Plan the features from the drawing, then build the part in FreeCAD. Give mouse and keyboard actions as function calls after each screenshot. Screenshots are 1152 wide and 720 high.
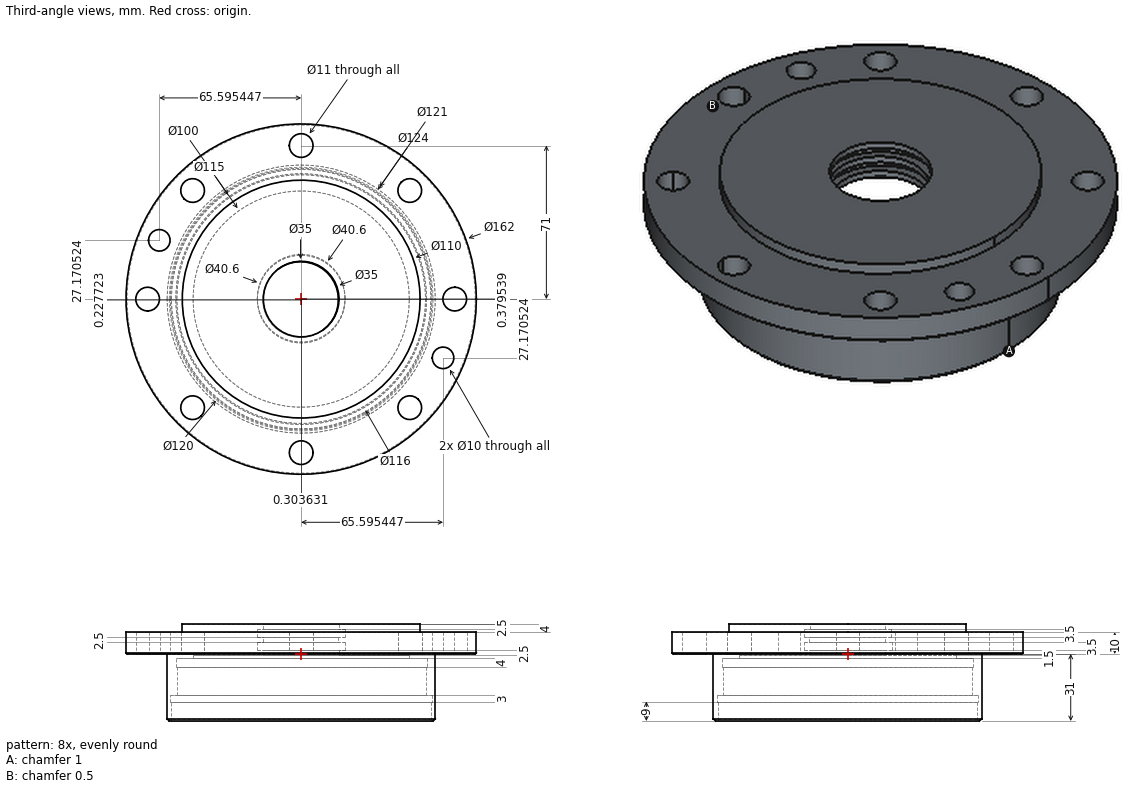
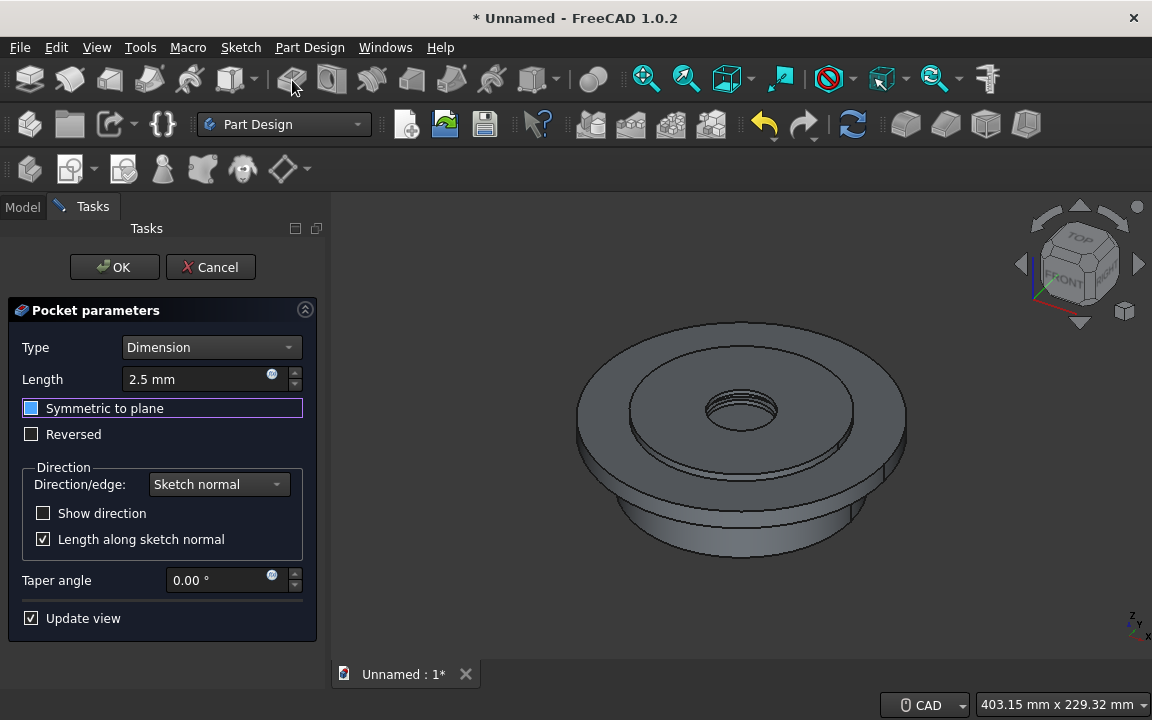
click(115, 267)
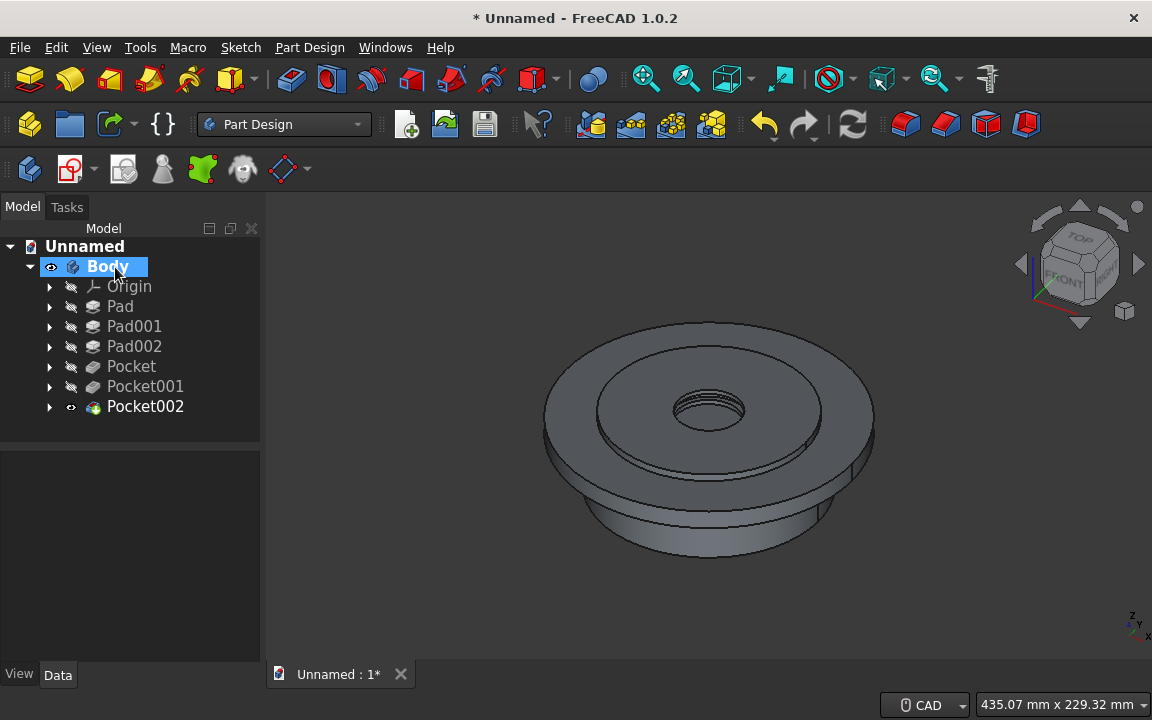
click(713, 418)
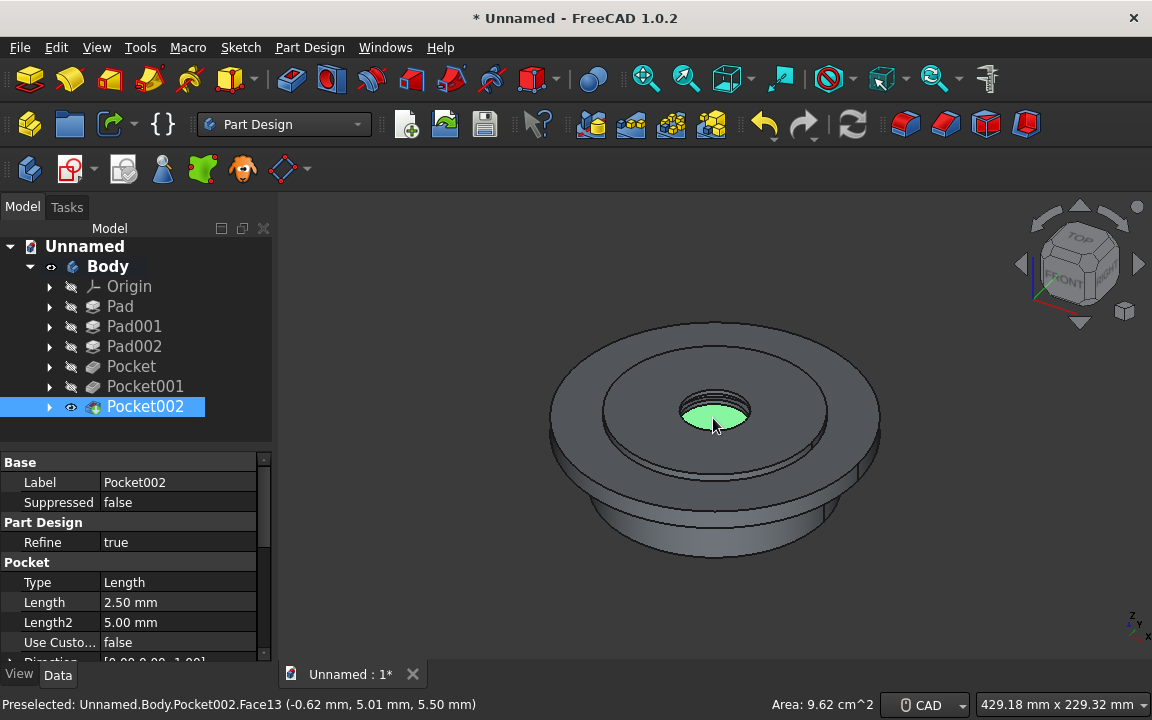
click(70, 170)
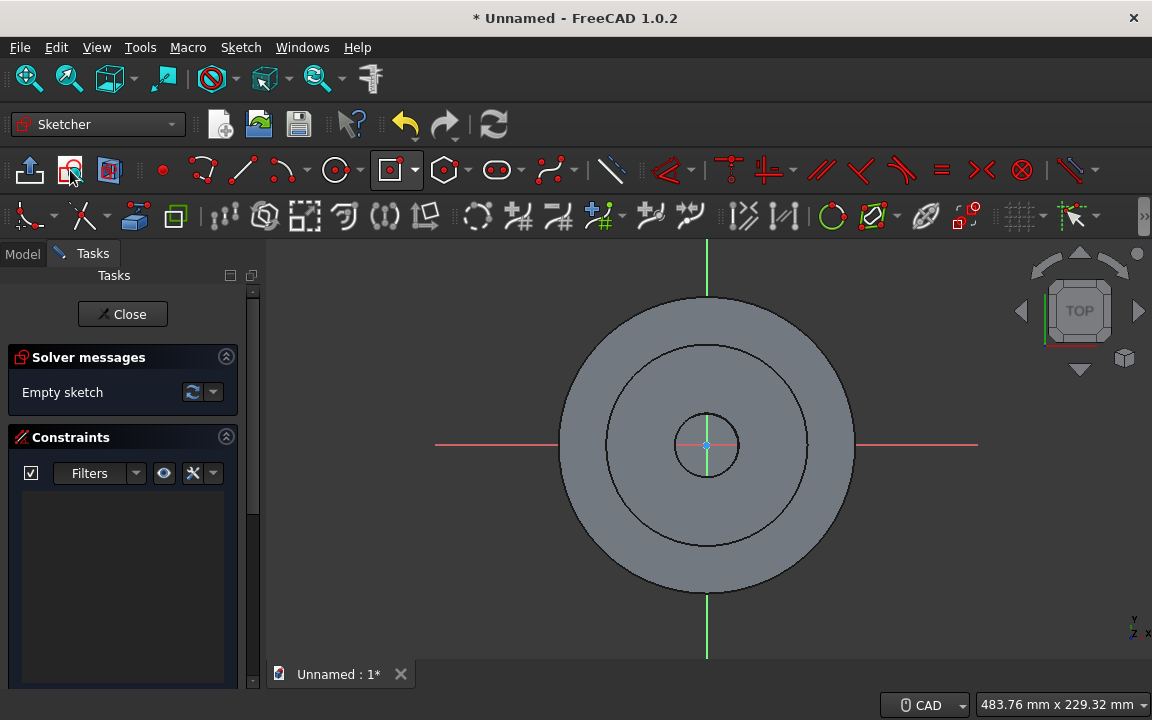
scroll(735, 443, up, 6)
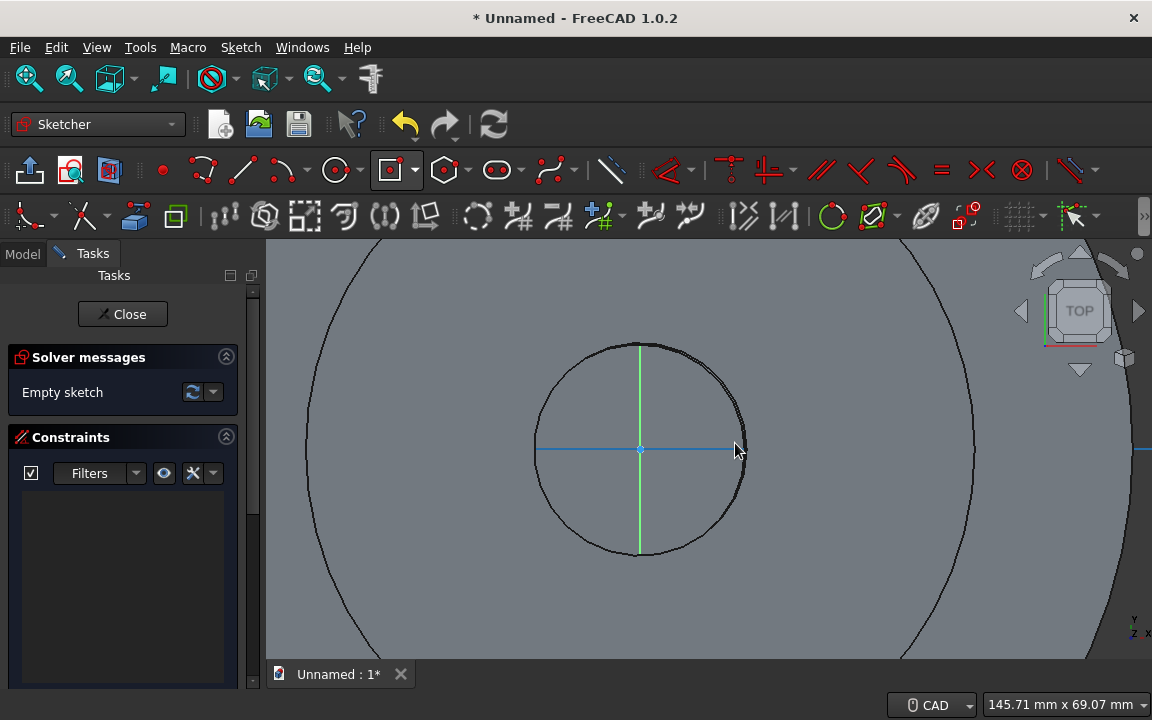
click(336, 170)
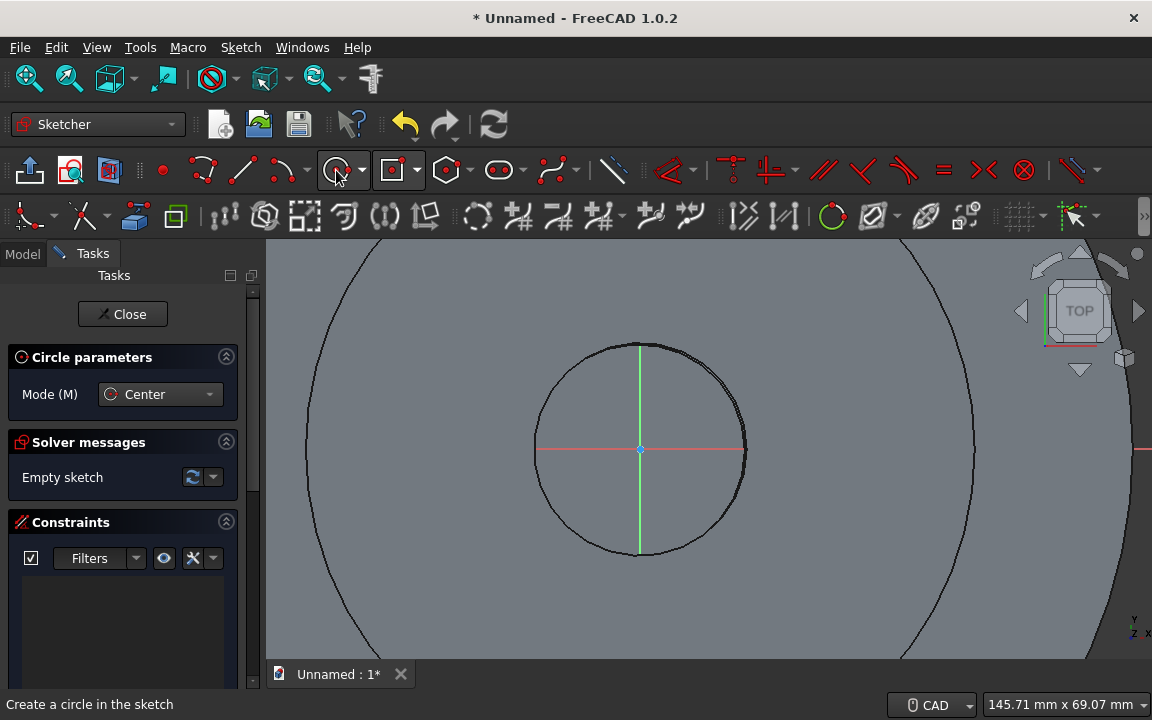
scroll(640, 447, up, 10)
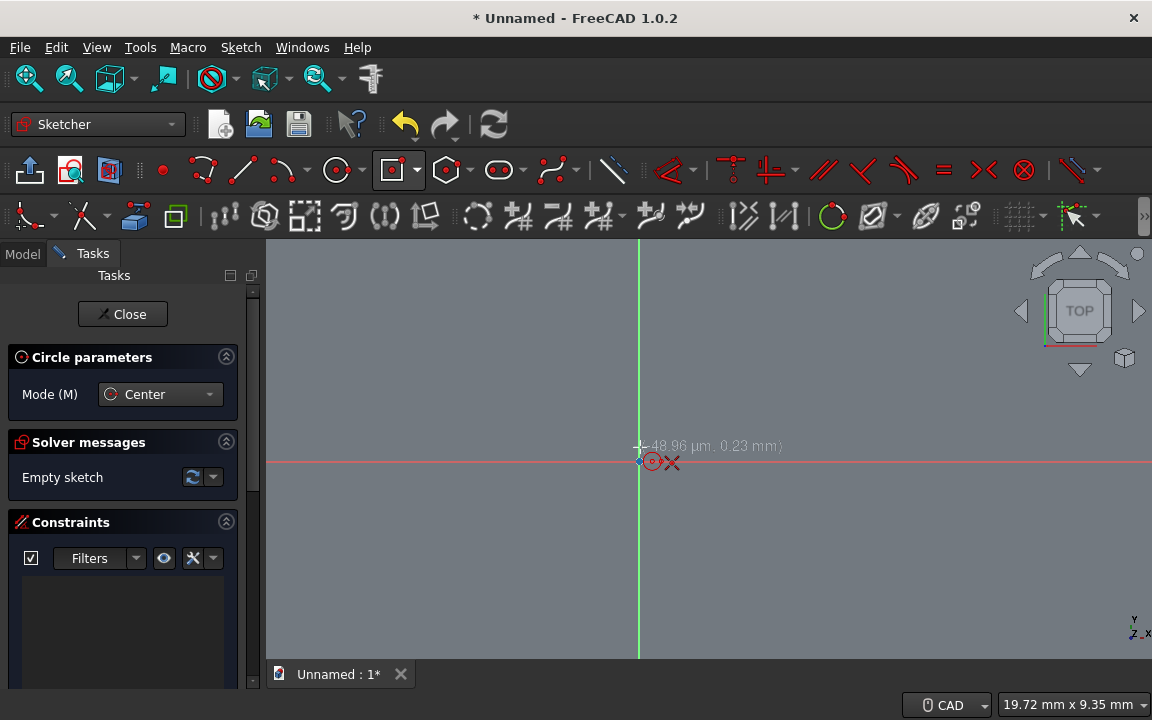
click(639, 445)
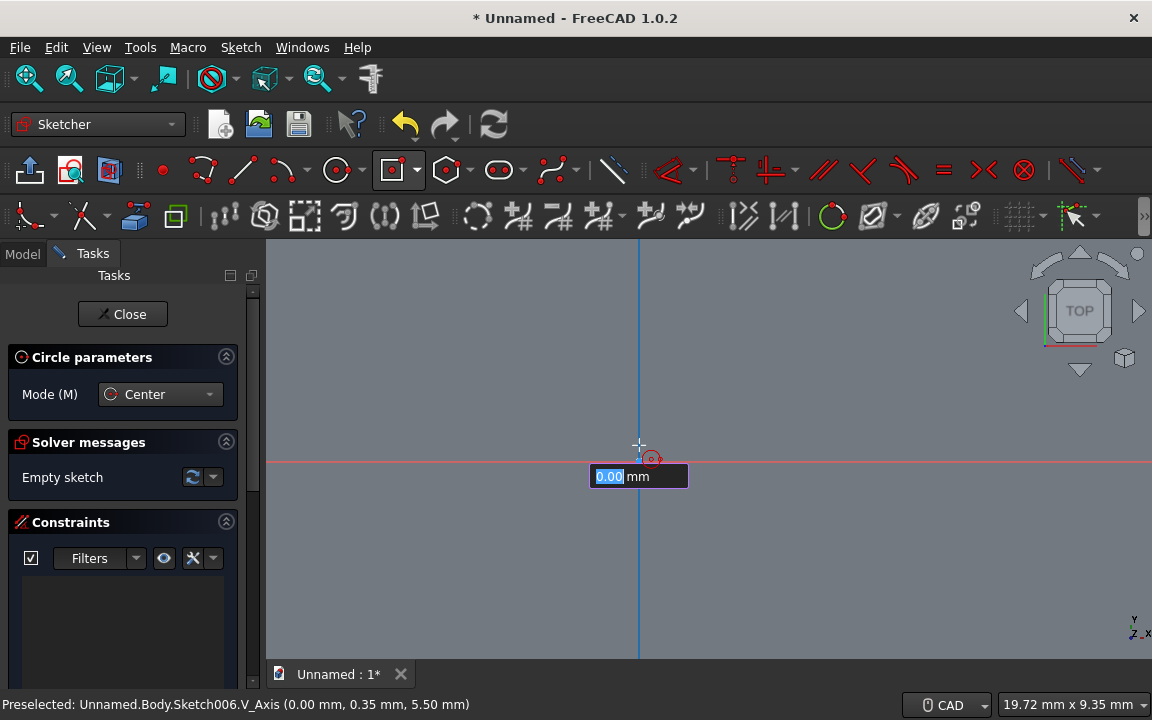
scroll(641, 450, down, 10)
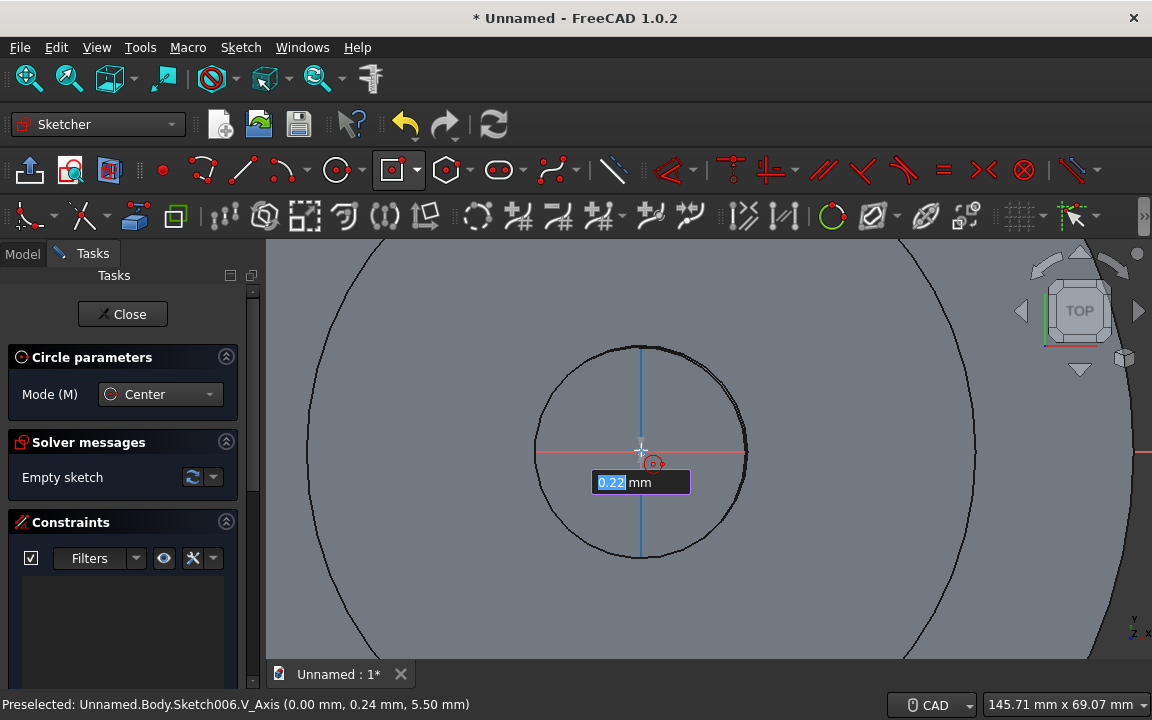
click(728, 362)
key(Escape)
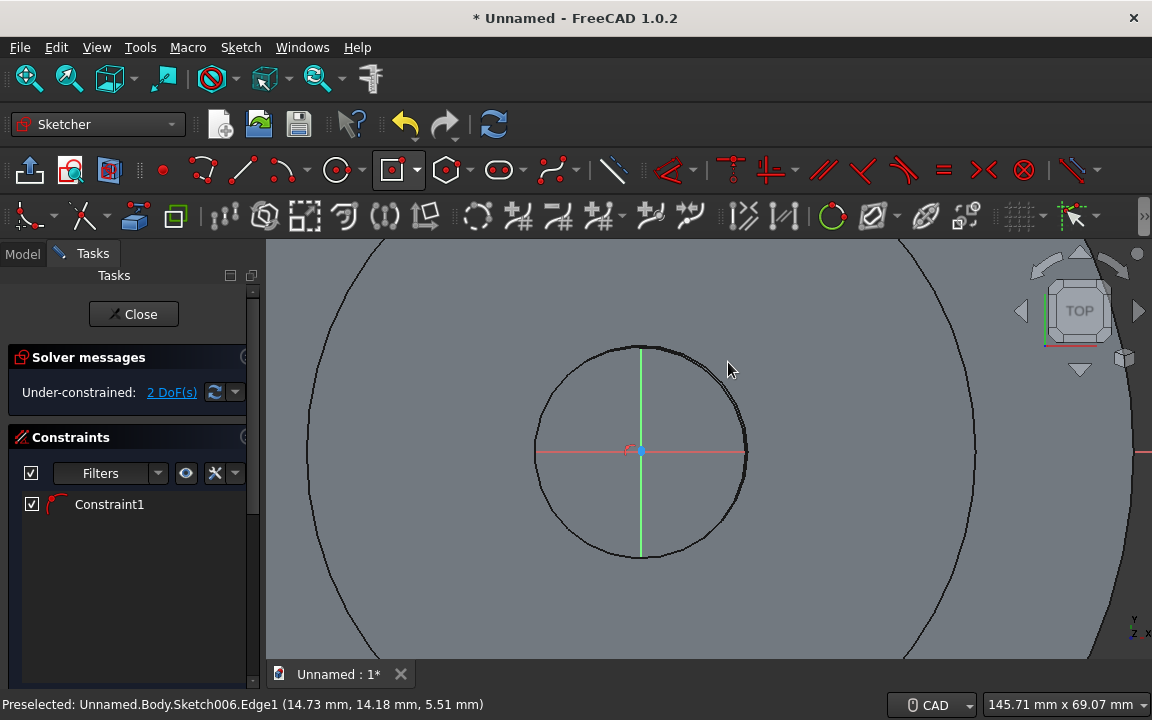
key(d)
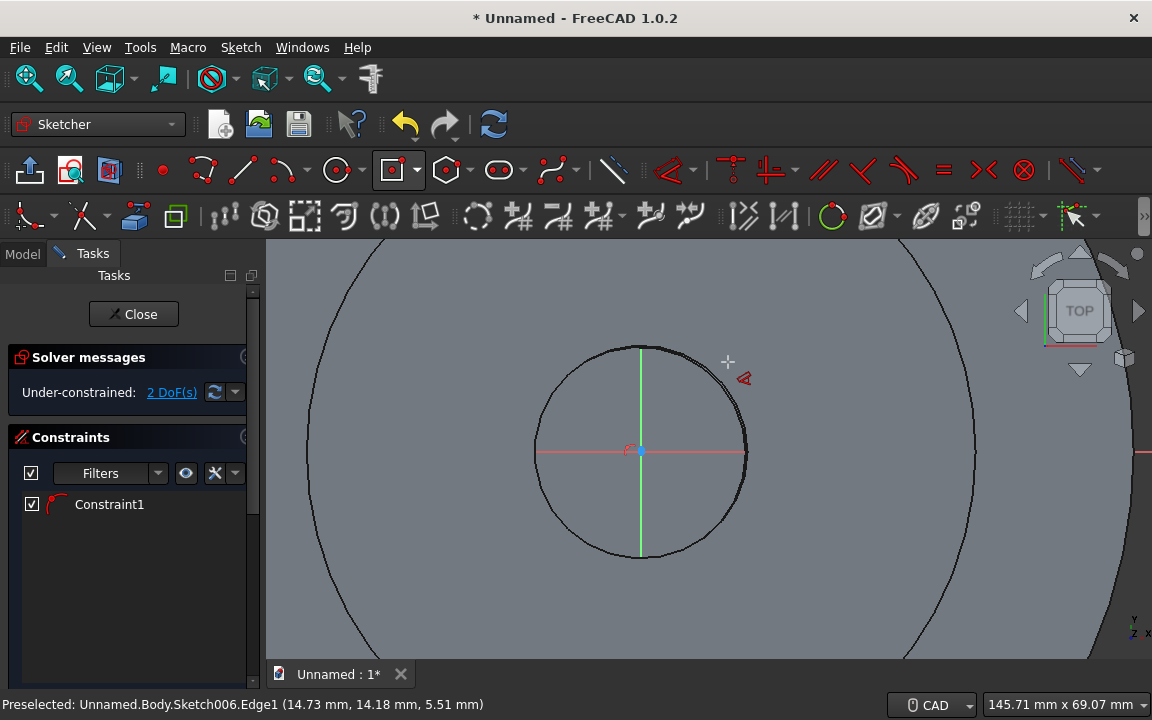
click(728, 363)
click(751, 340)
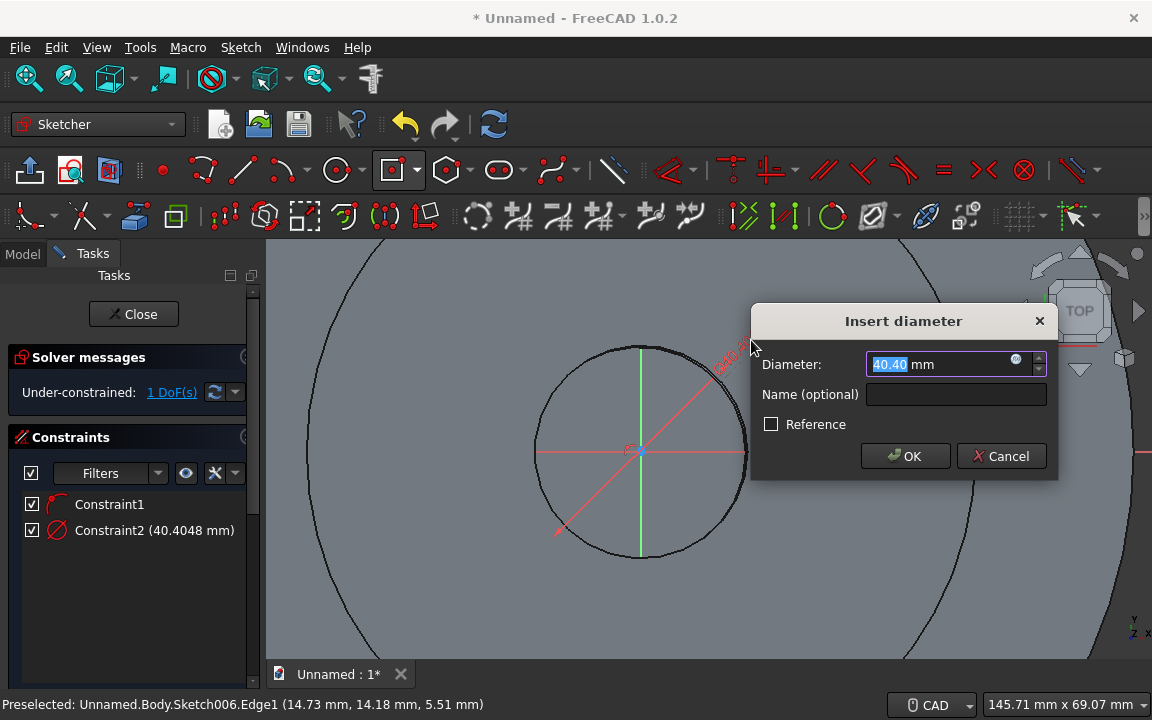
text(40.6)
key(Return)